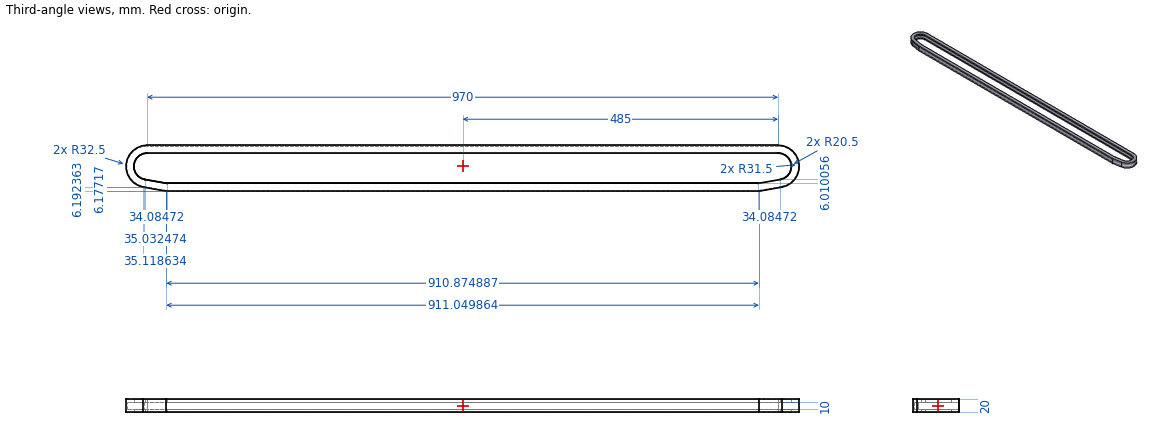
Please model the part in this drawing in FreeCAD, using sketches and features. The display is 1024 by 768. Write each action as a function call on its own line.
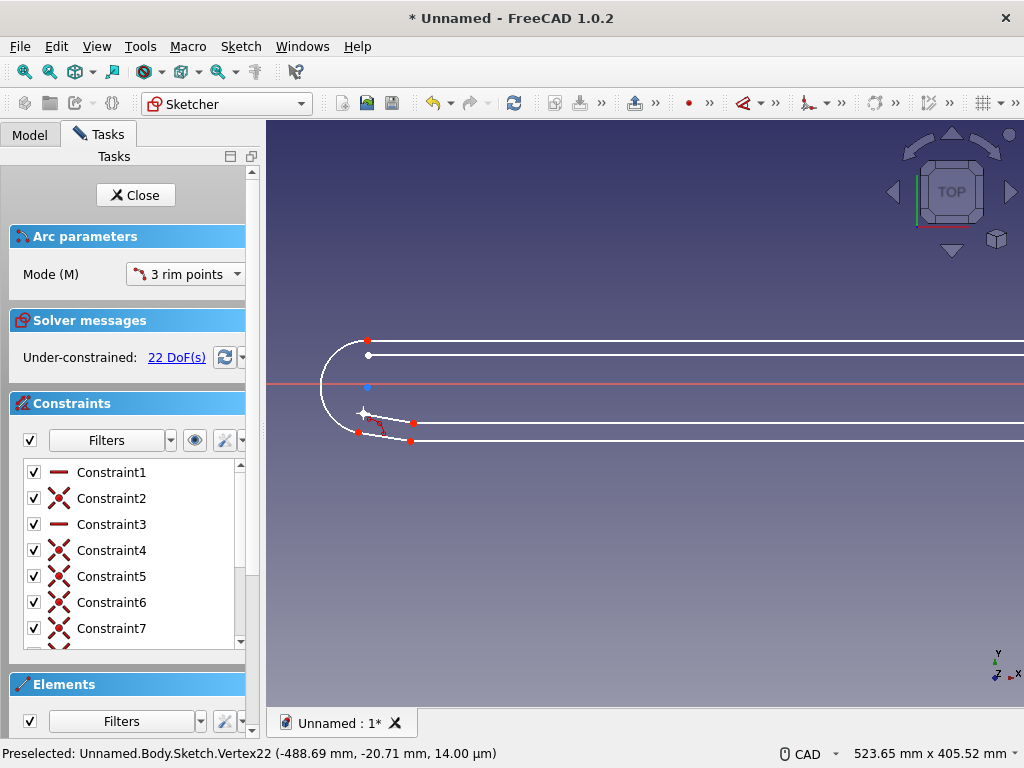
scroll(415, 422, down, 7)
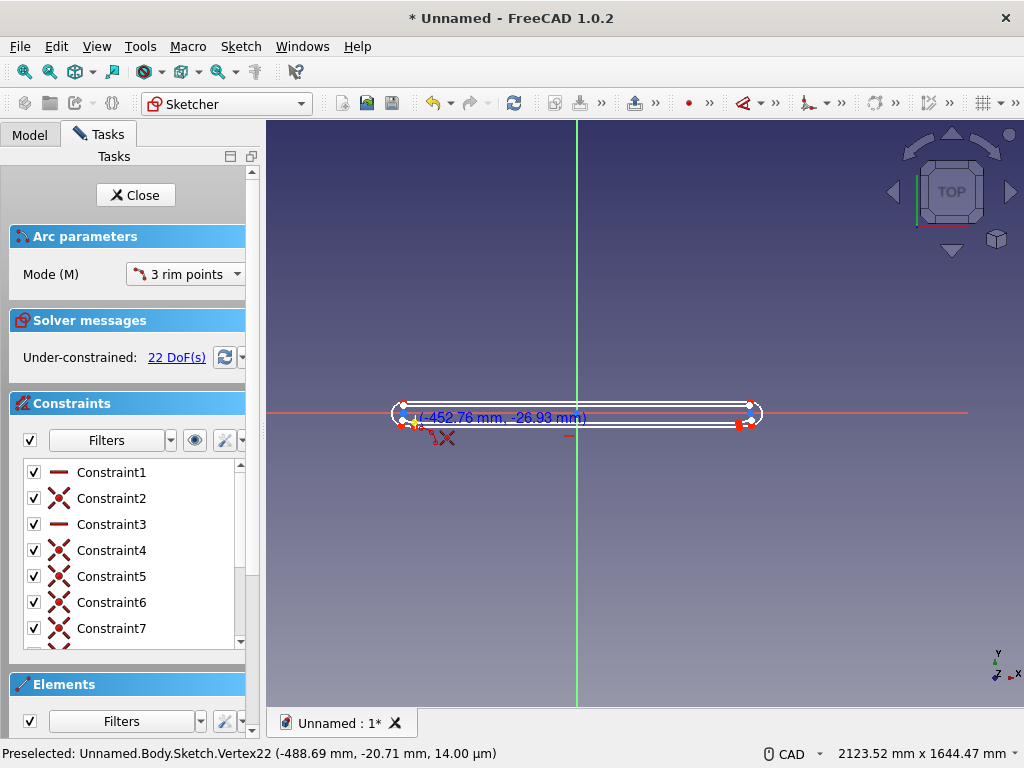
scroll(750, 406, up, 7)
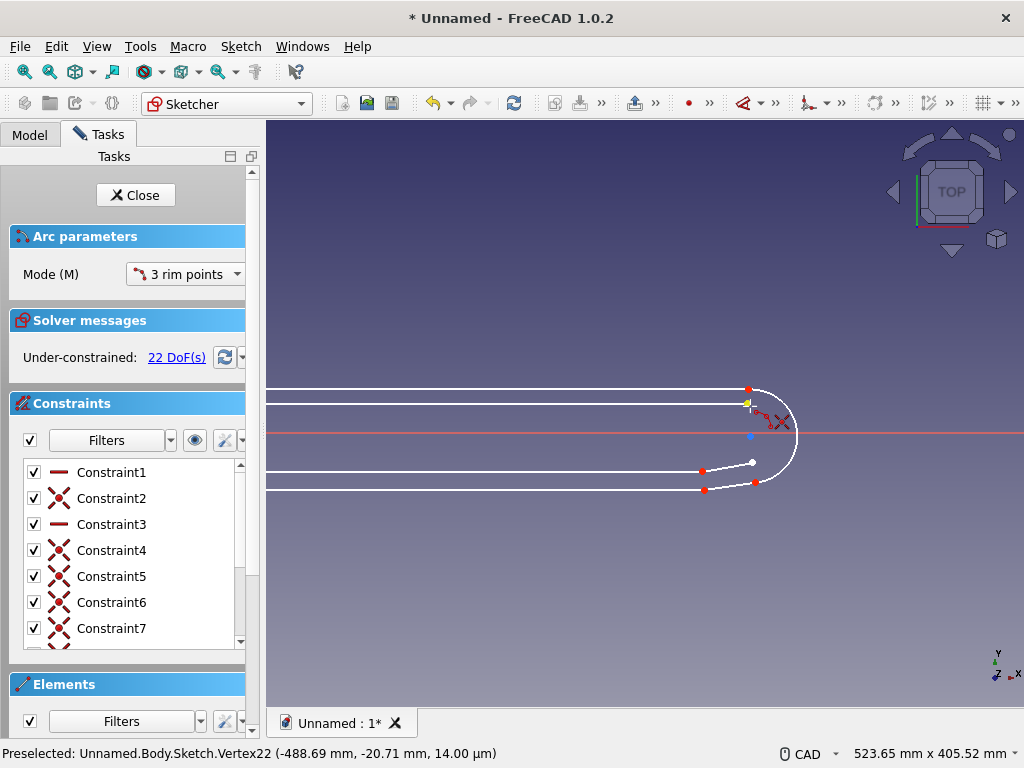
click(748, 404)
click(753, 463)
click(771, 414)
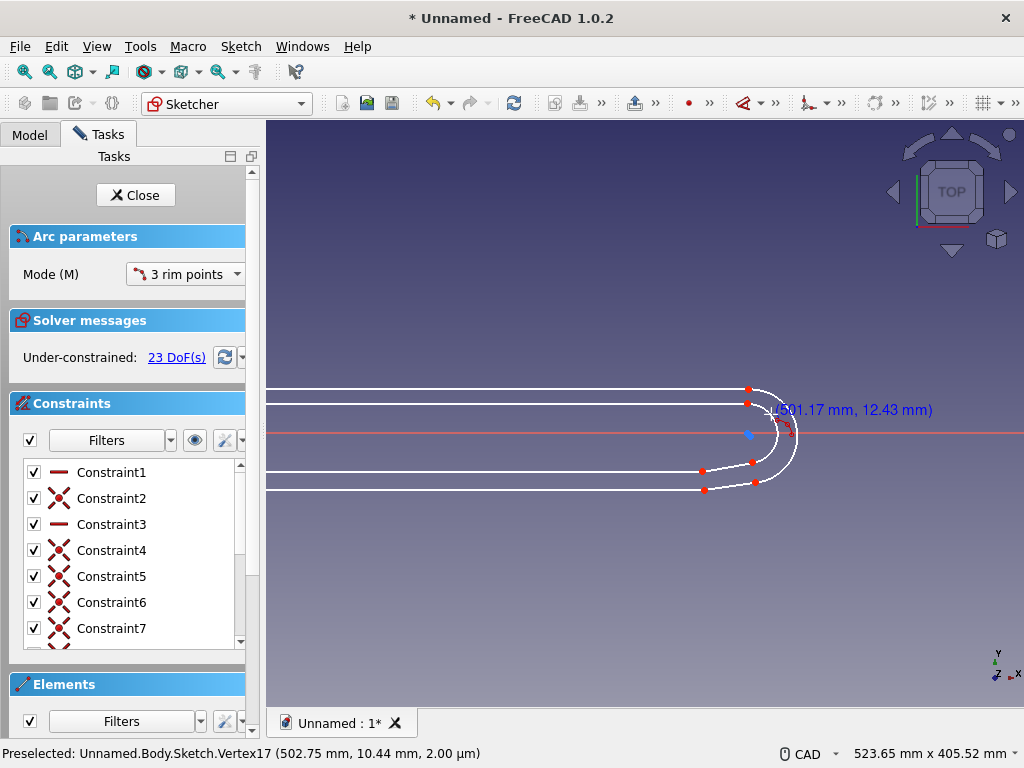
scroll(750, 406, down, 7)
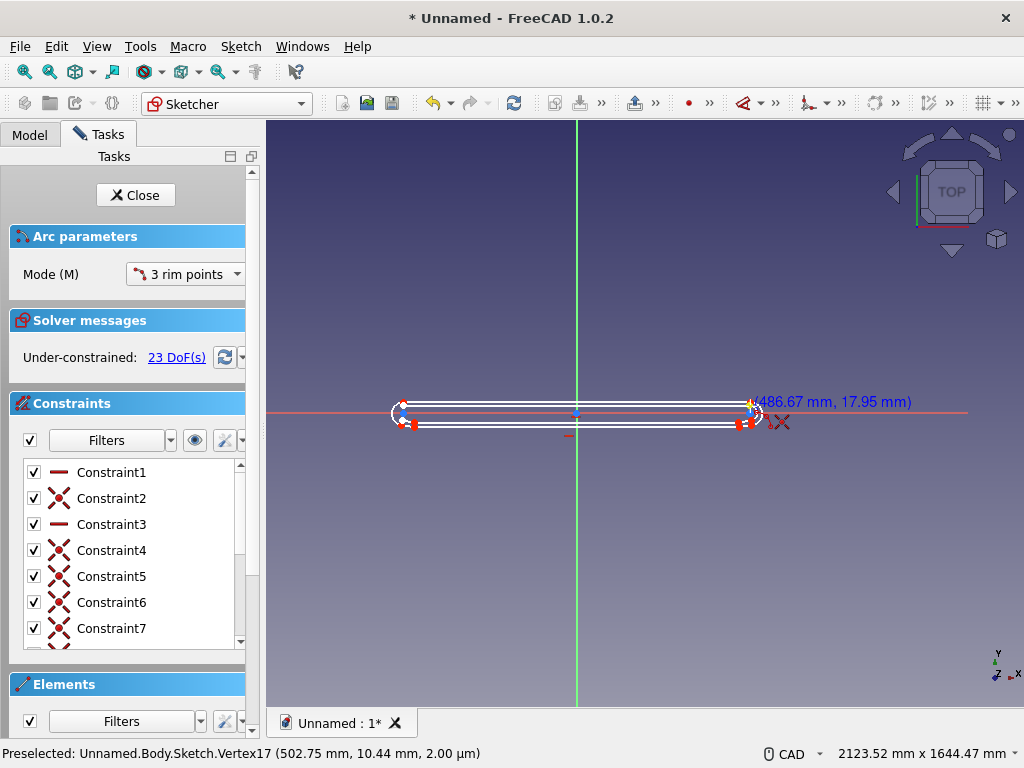
scroll(402, 420, up, 7)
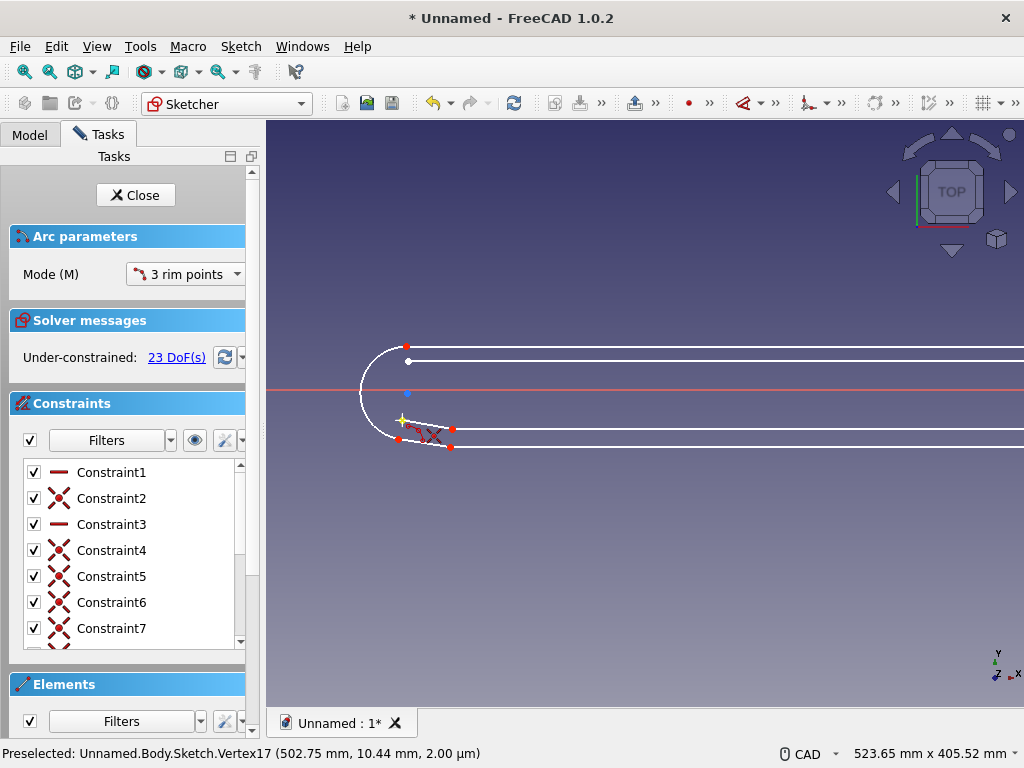
click(403, 420)
click(408, 361)
click(385, 371)
key(Escape)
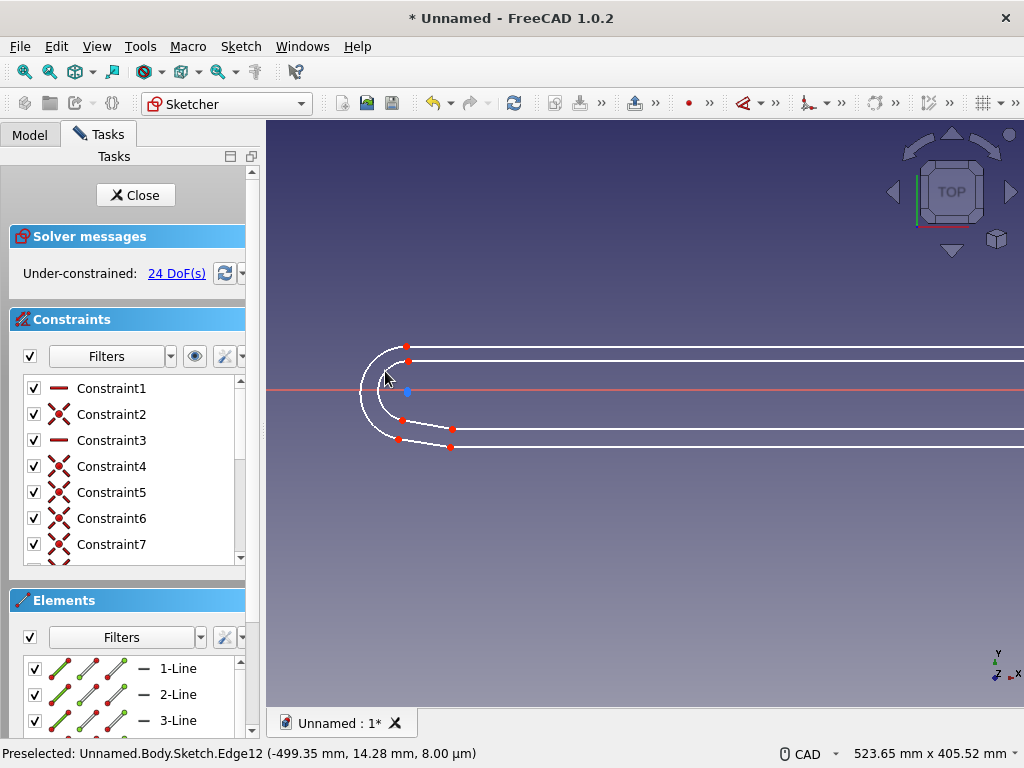
click(829, 347)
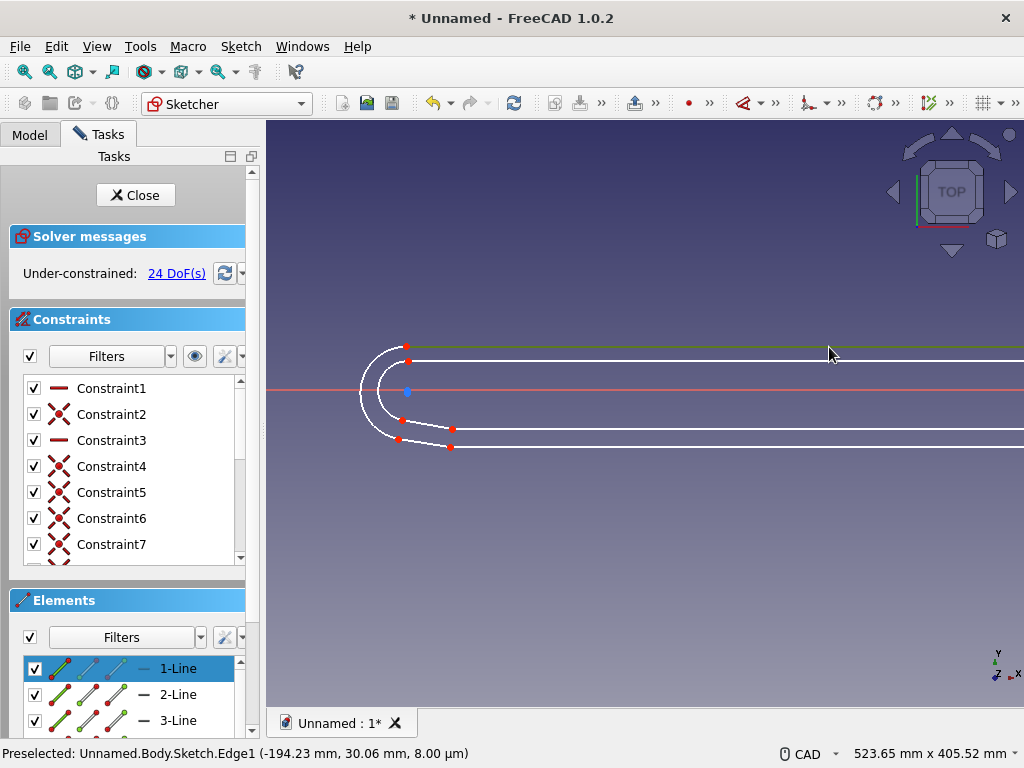
click(371, 364)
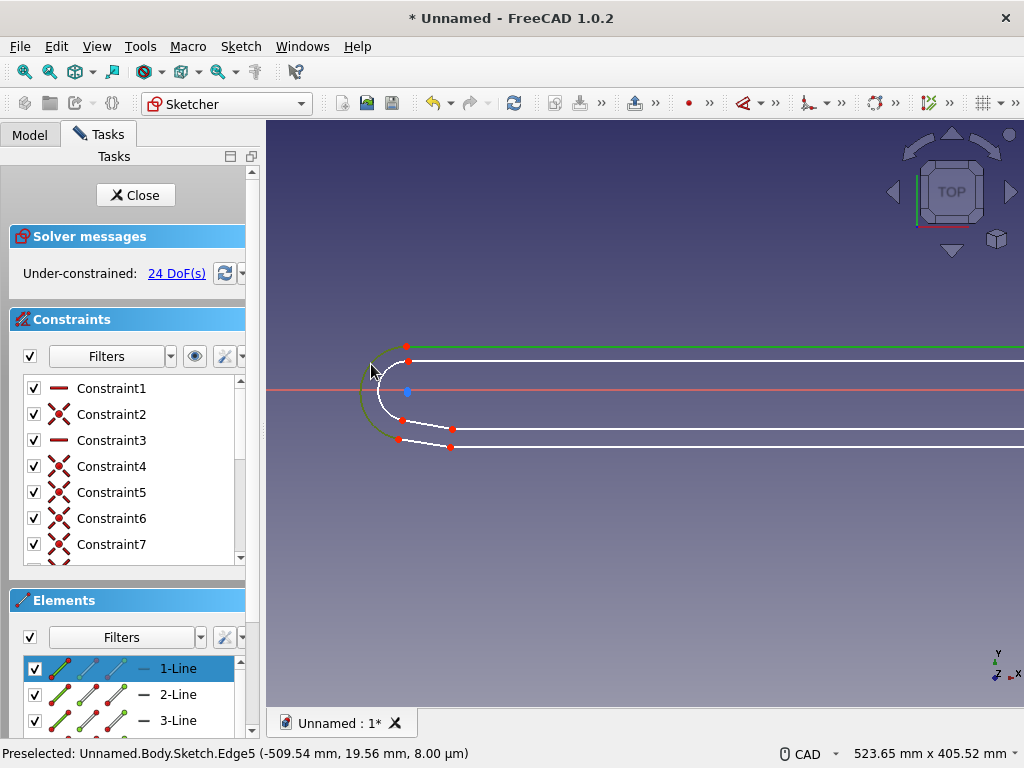
key(t)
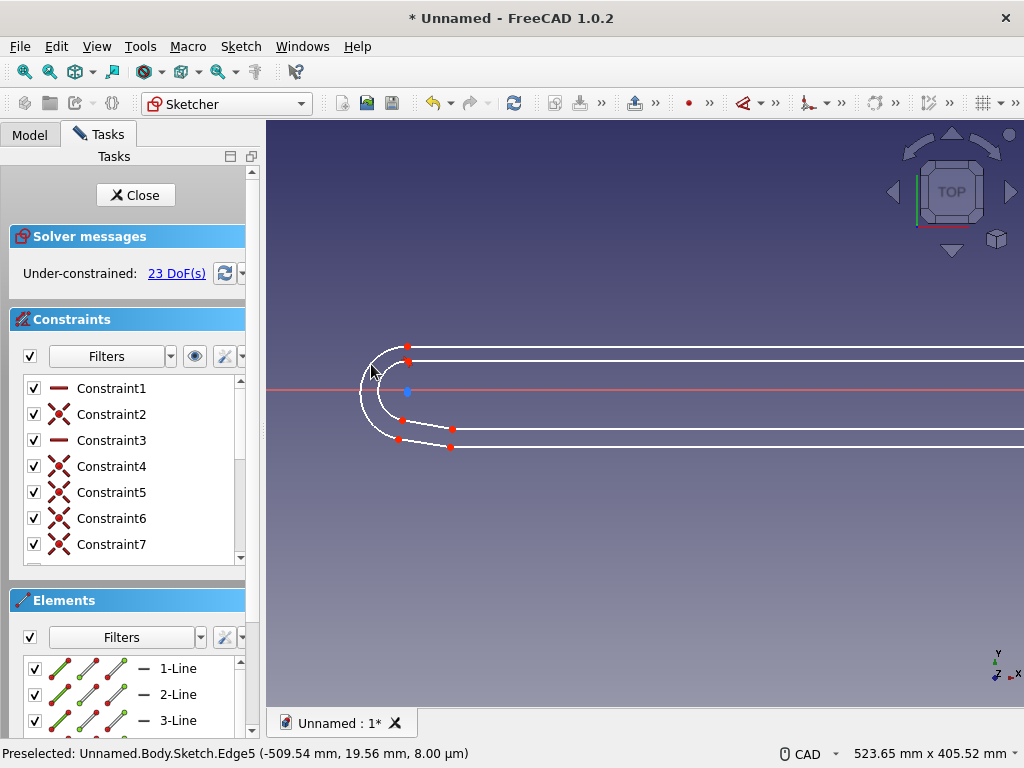
click(829, 347)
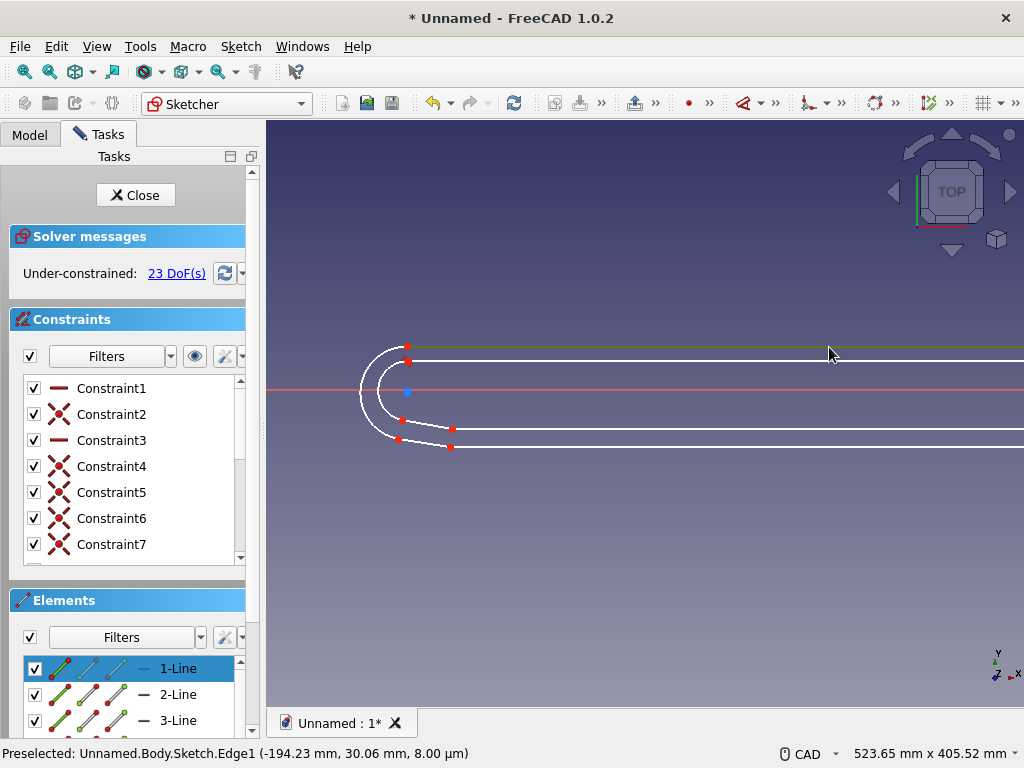
scroll(402, 420, down, 7)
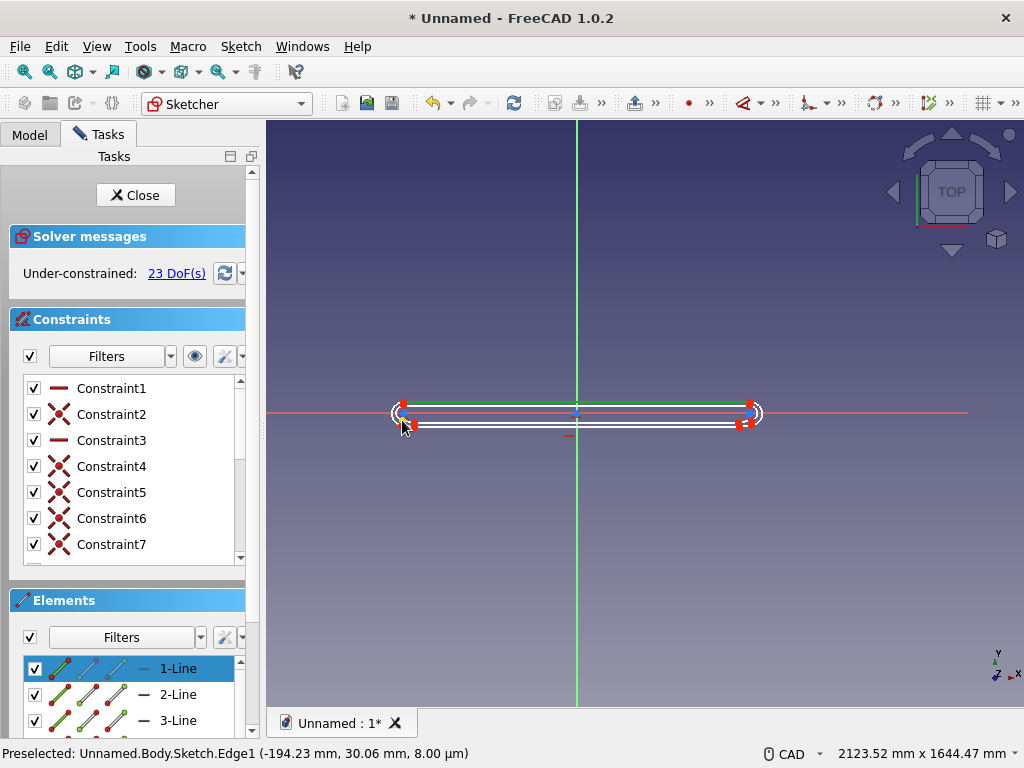
scroll(760, 420, up, 5)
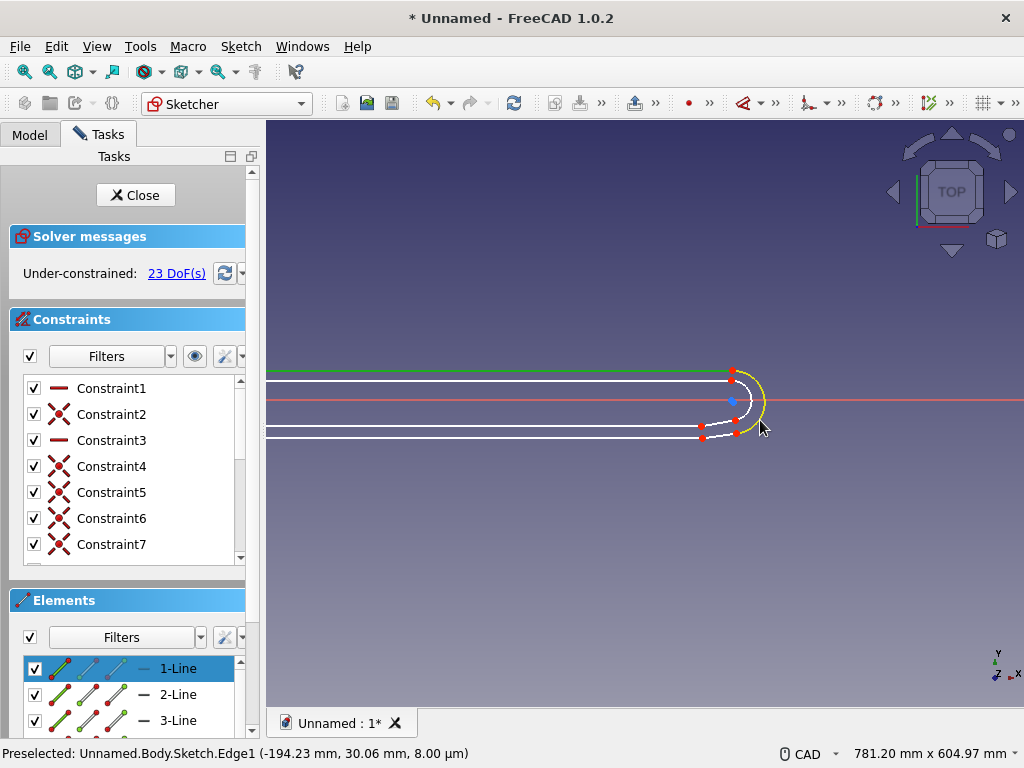
click(760, 419)